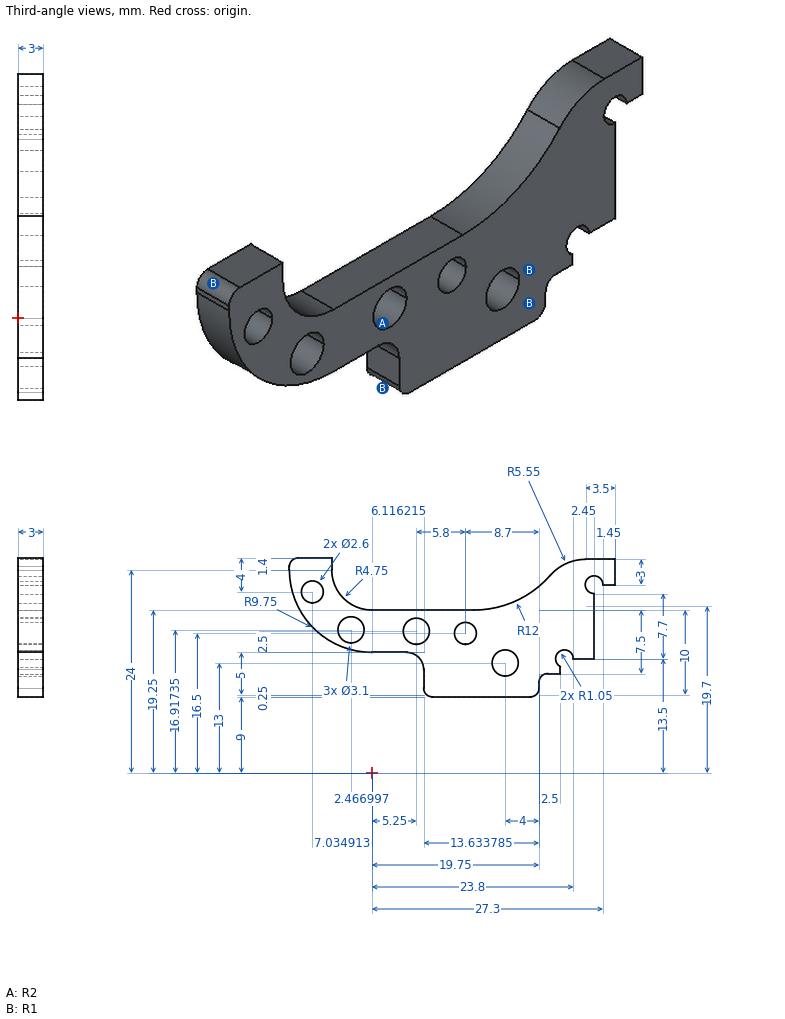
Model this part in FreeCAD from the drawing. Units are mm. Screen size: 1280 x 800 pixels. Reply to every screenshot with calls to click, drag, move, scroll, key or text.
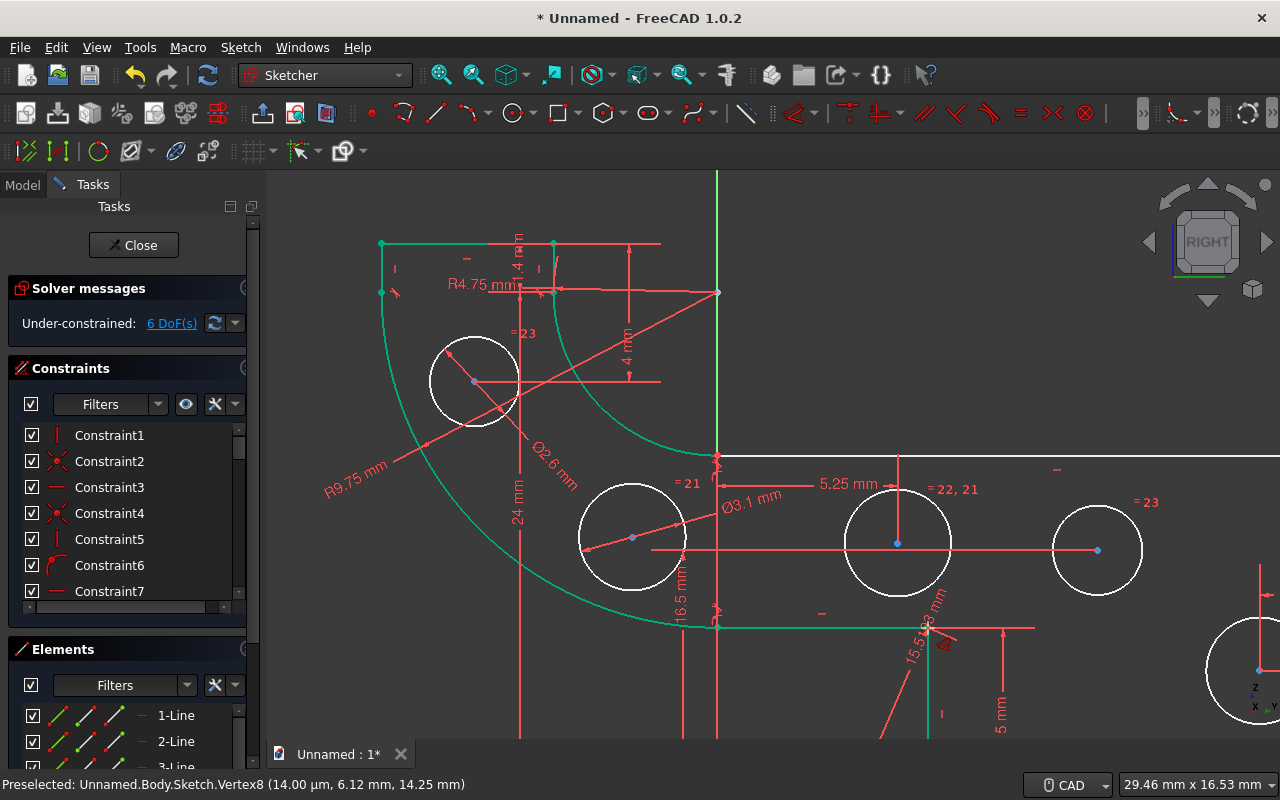
click(898, 543)
click(962, 585)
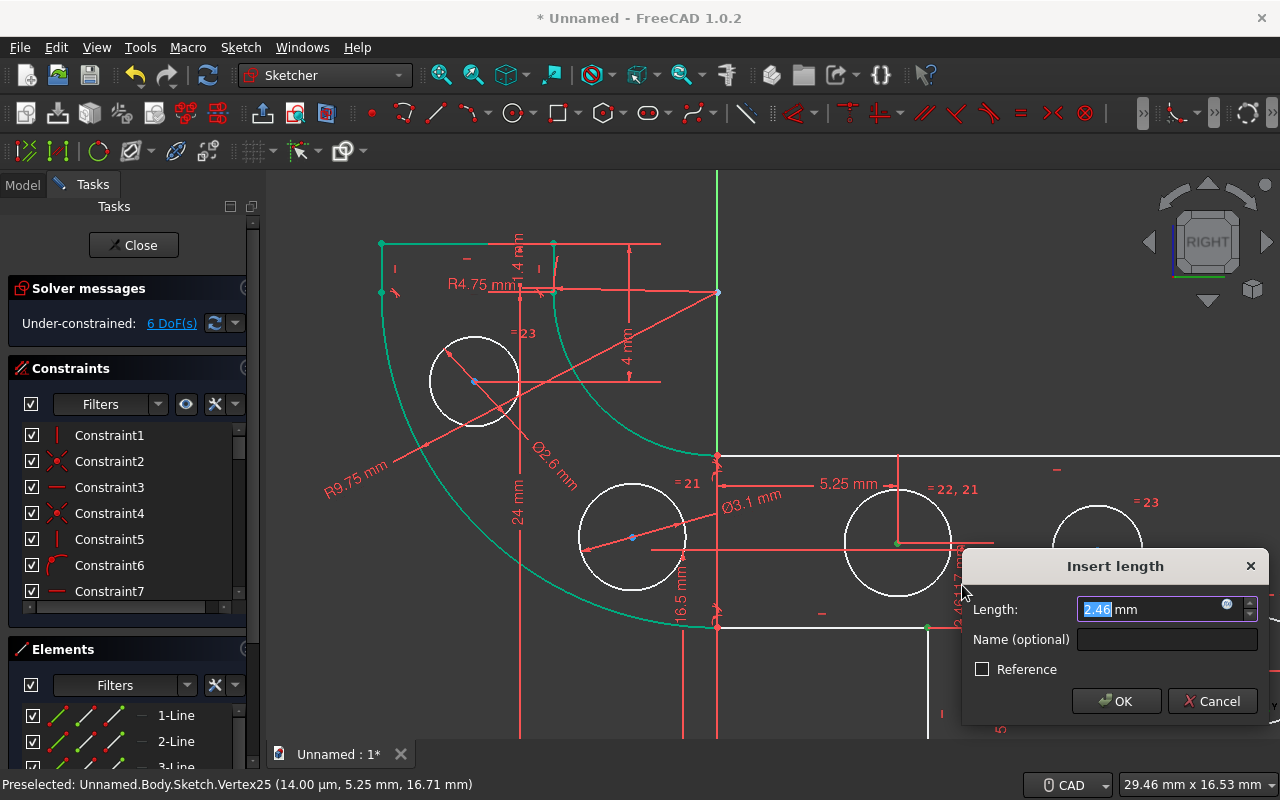
text(2.5)
key(Return)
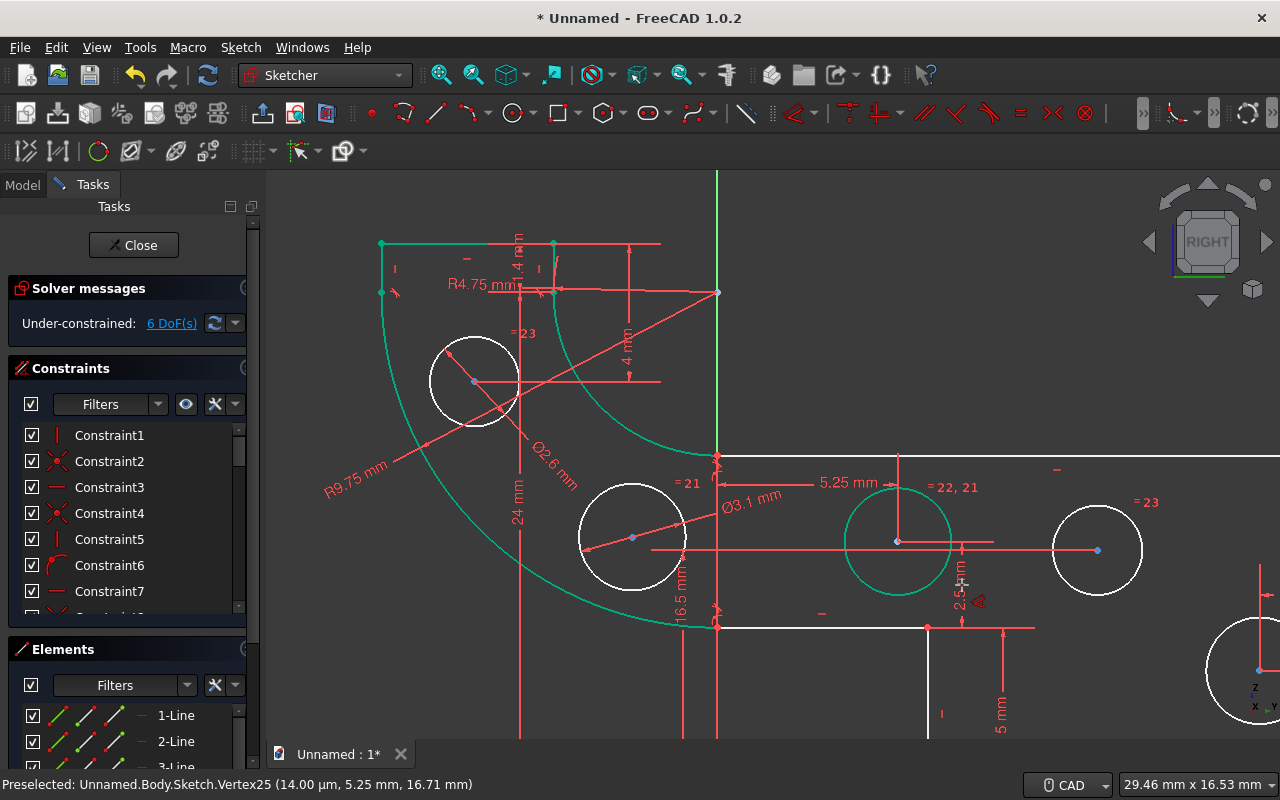
click(898, 542)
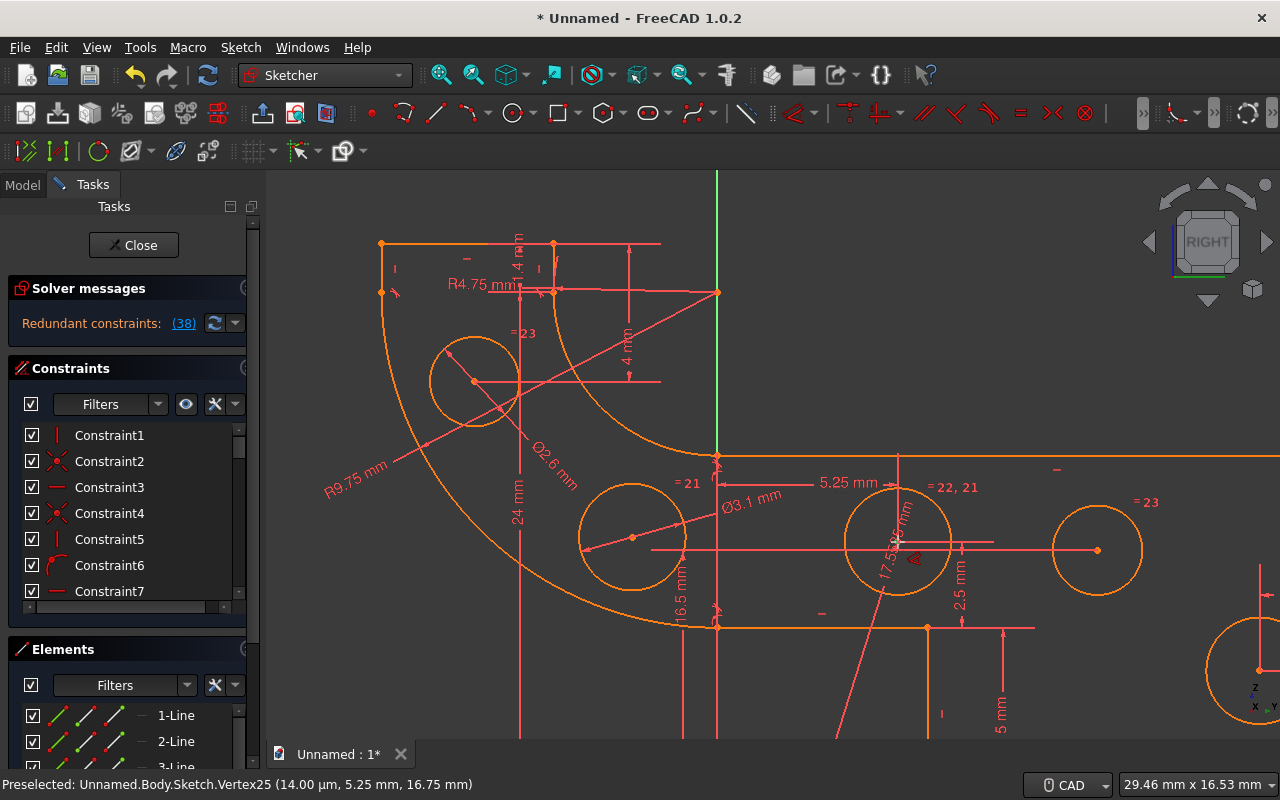
click(1098, 550)
click(998, 508)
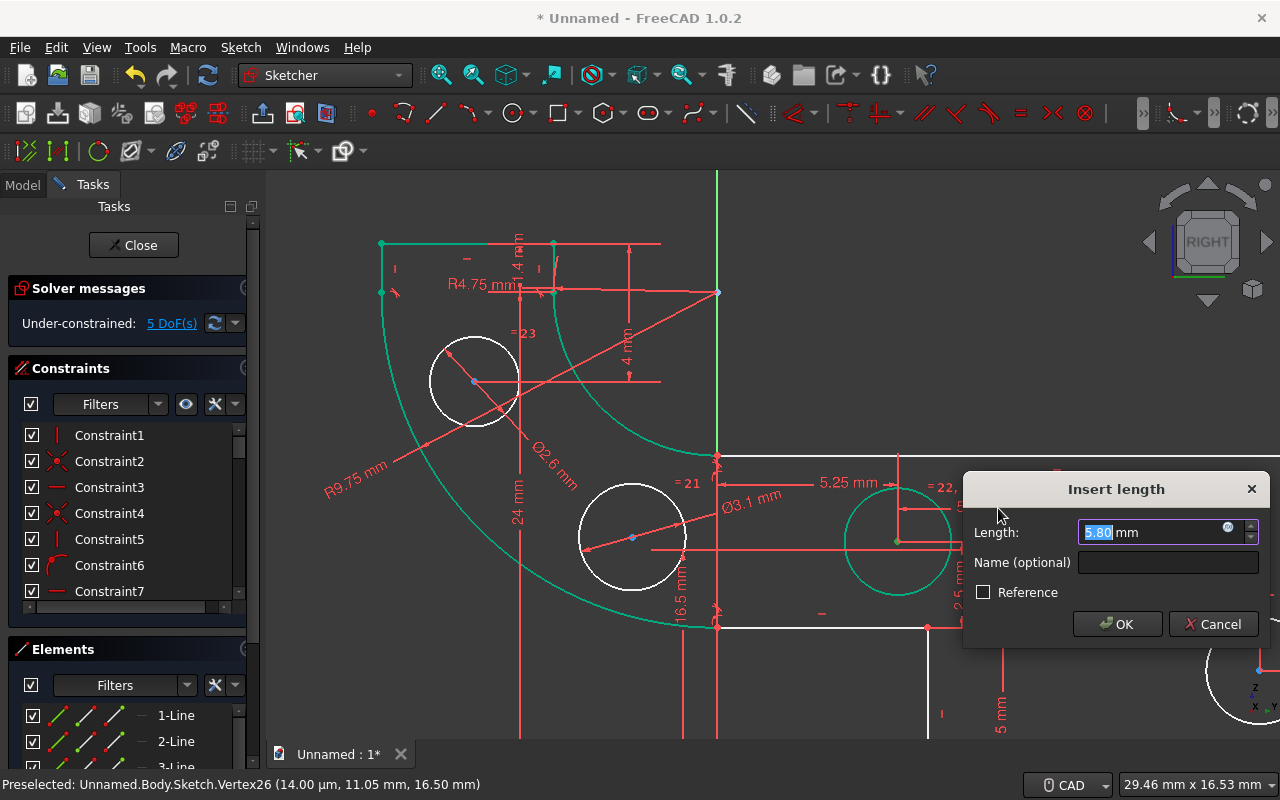
text(5.8)
key(Return)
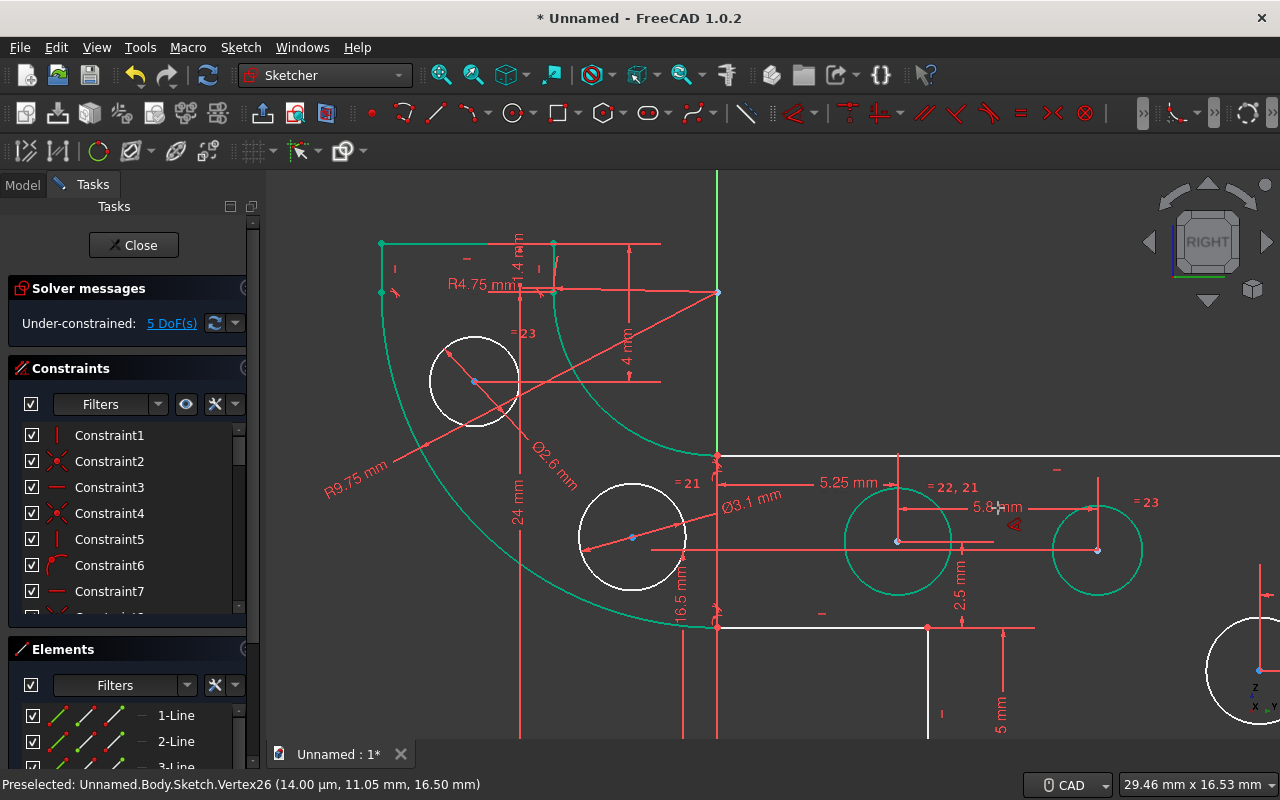
scroll(554, 270, down, 4)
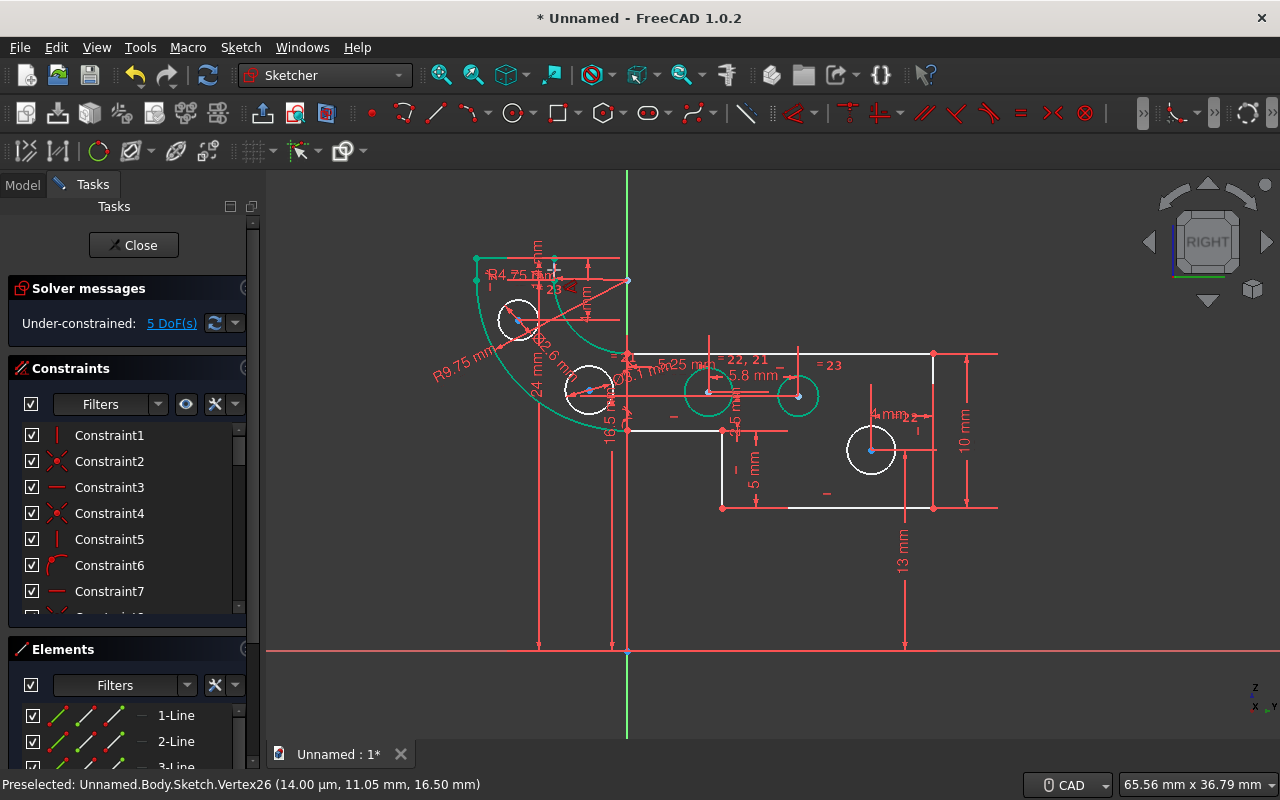
click(933, 354)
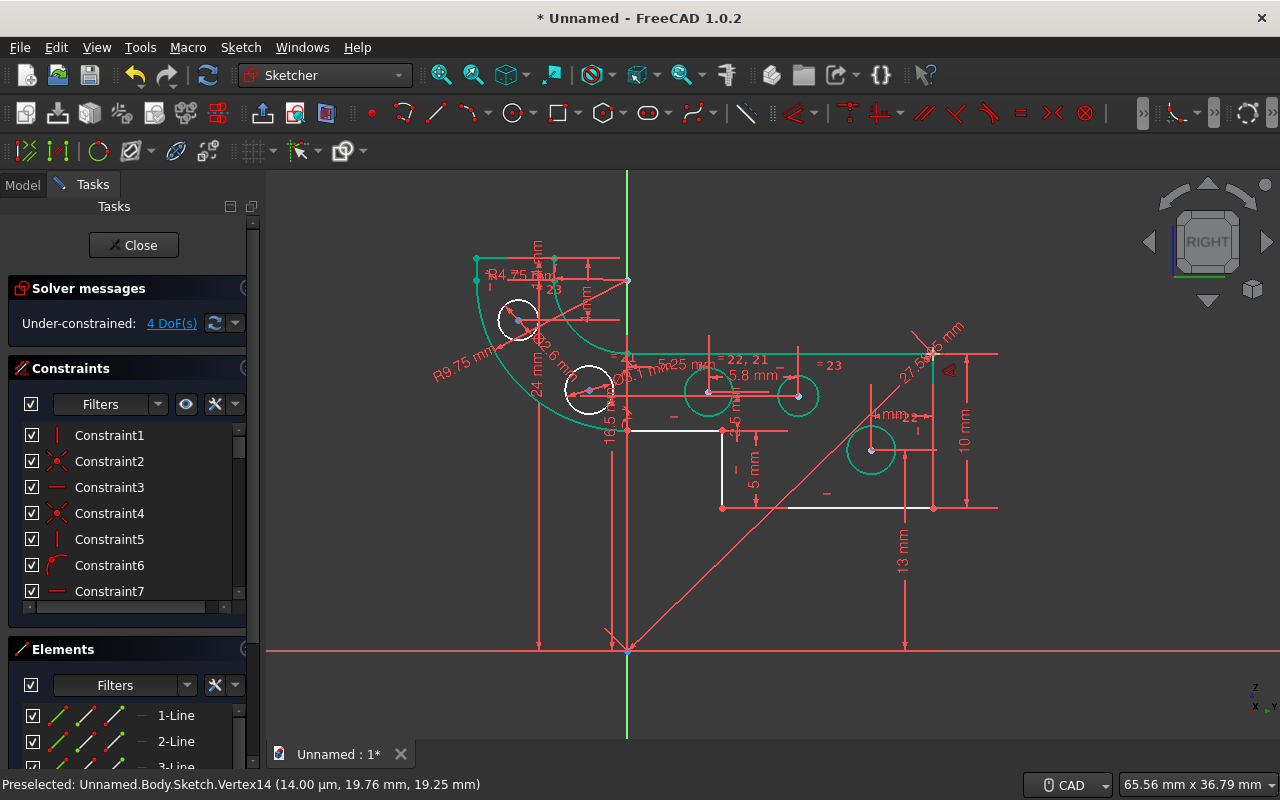
click(798, 396)
click(866, 320)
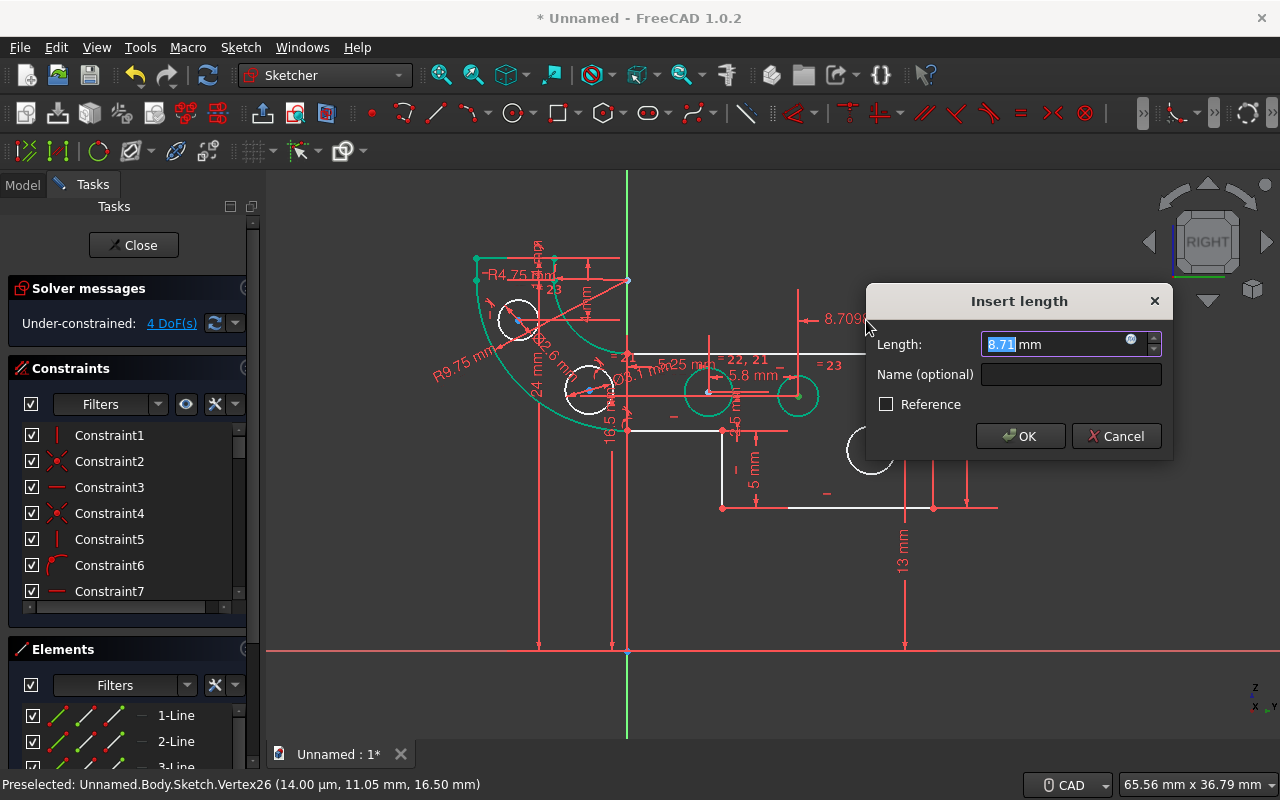
text(8.7)
key(Return)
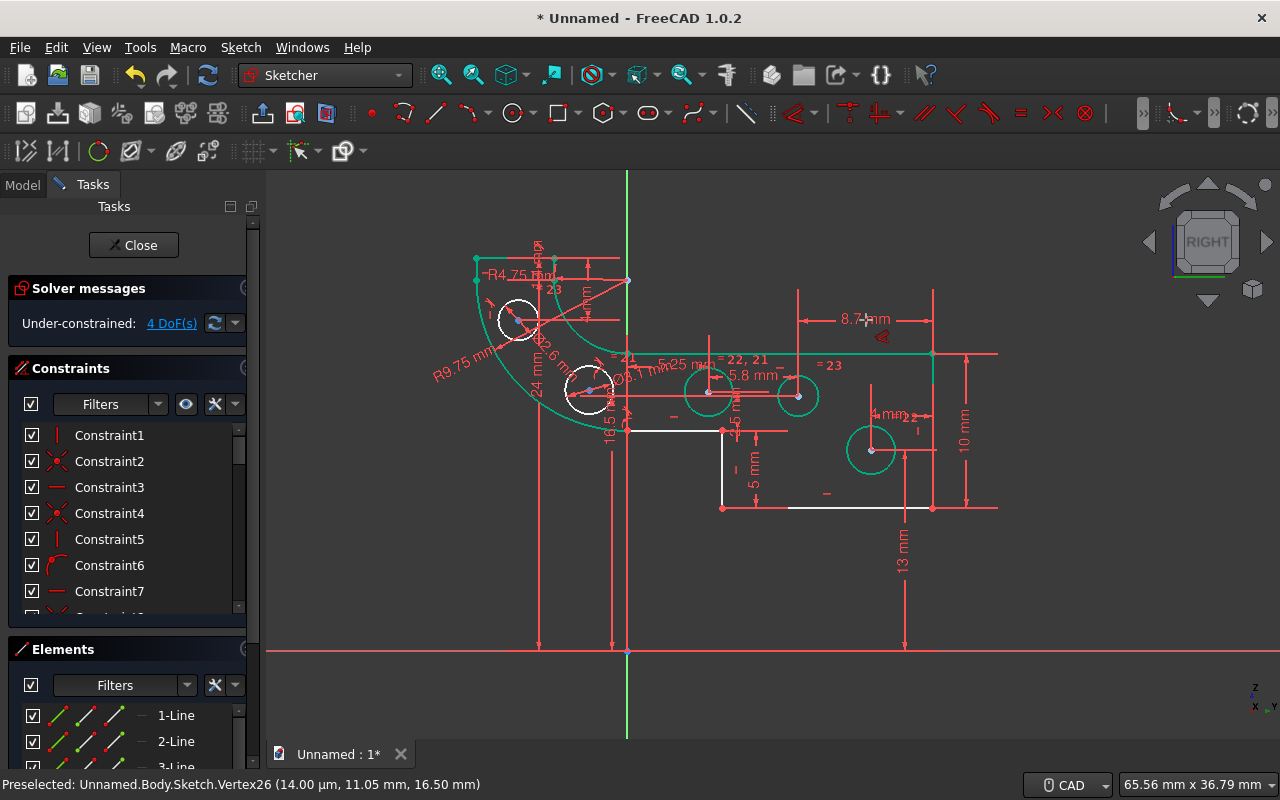
click(656, 431)
click(675, 465)